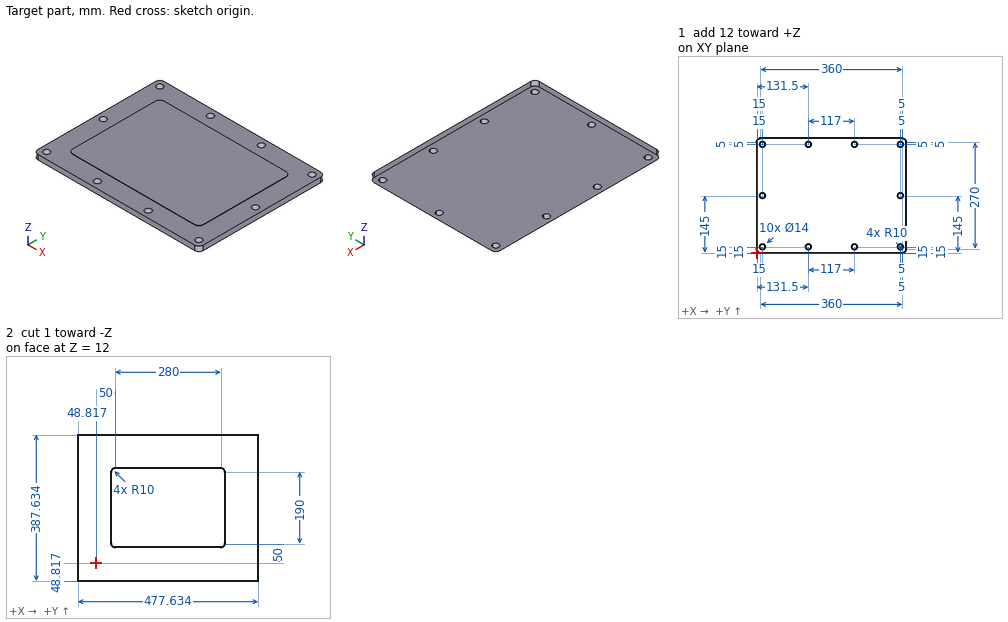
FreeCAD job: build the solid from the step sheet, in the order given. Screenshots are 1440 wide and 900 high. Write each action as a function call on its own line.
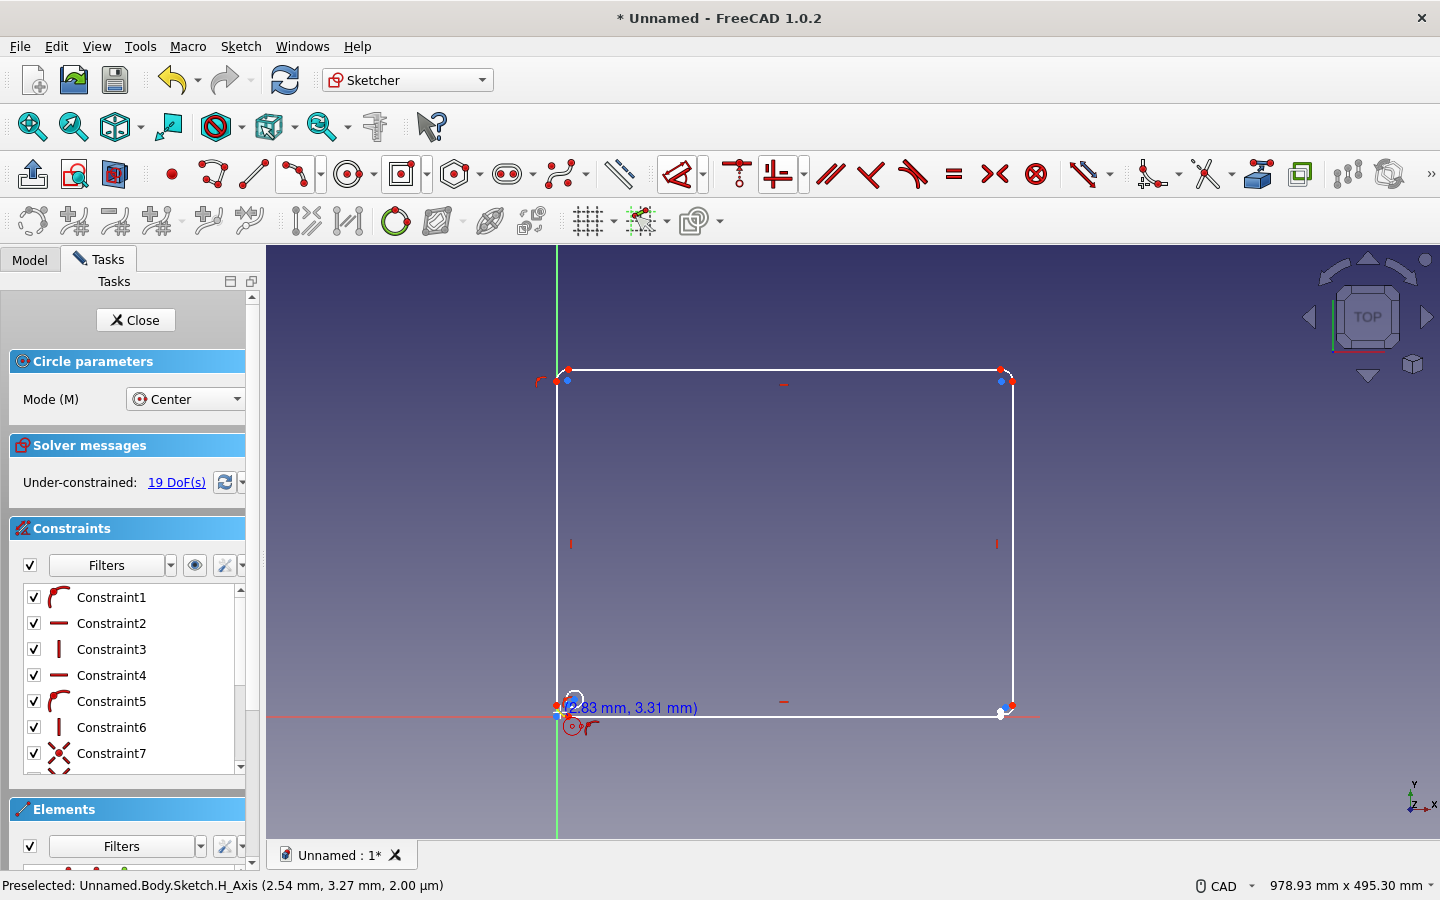
scroll(715, 699, up, 5)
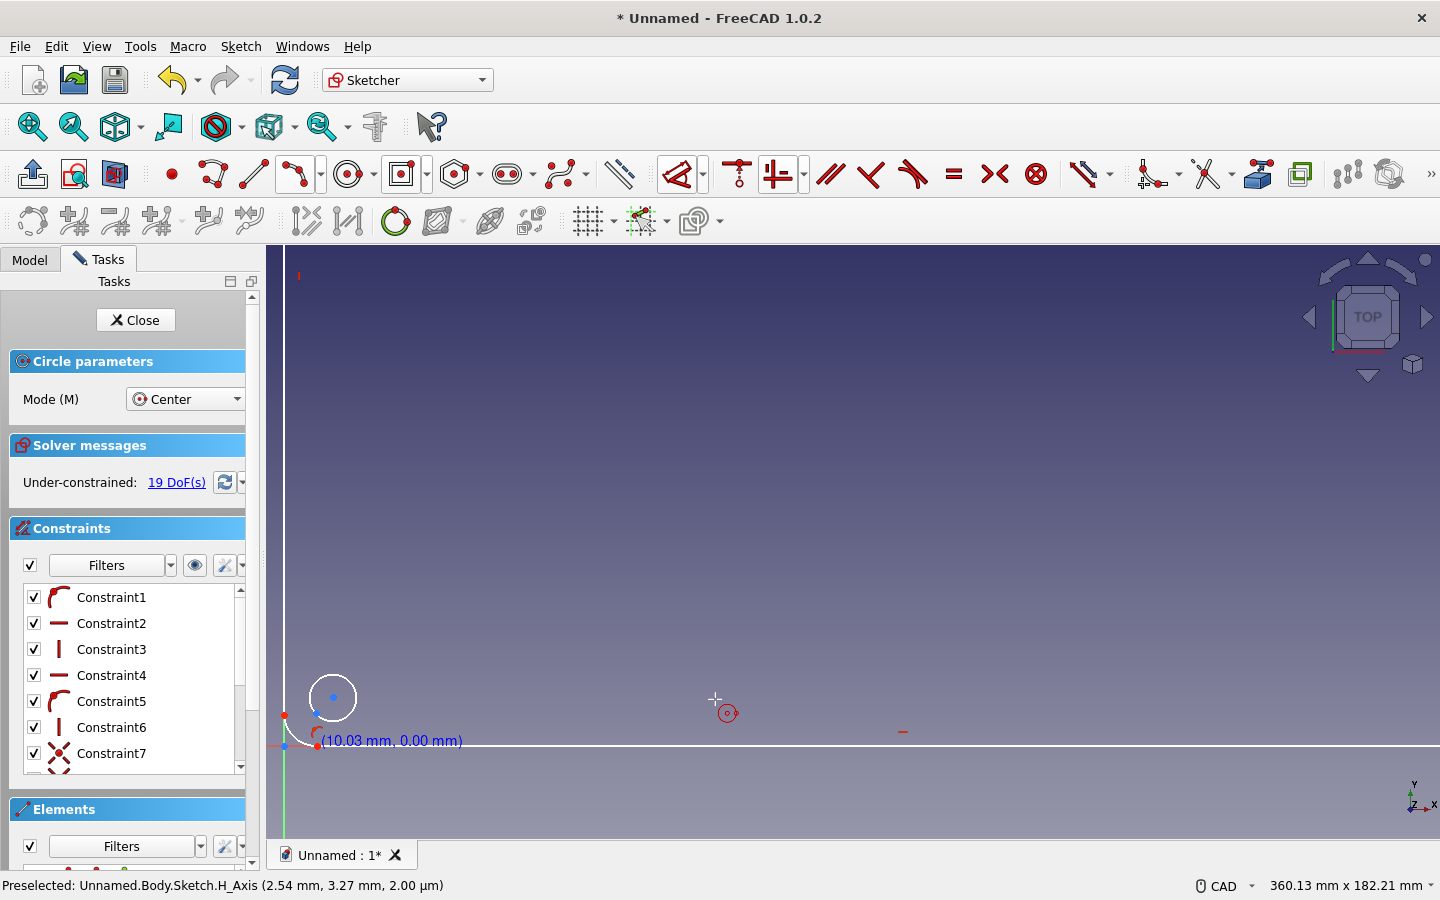
click(713, 697)
click(729, 681)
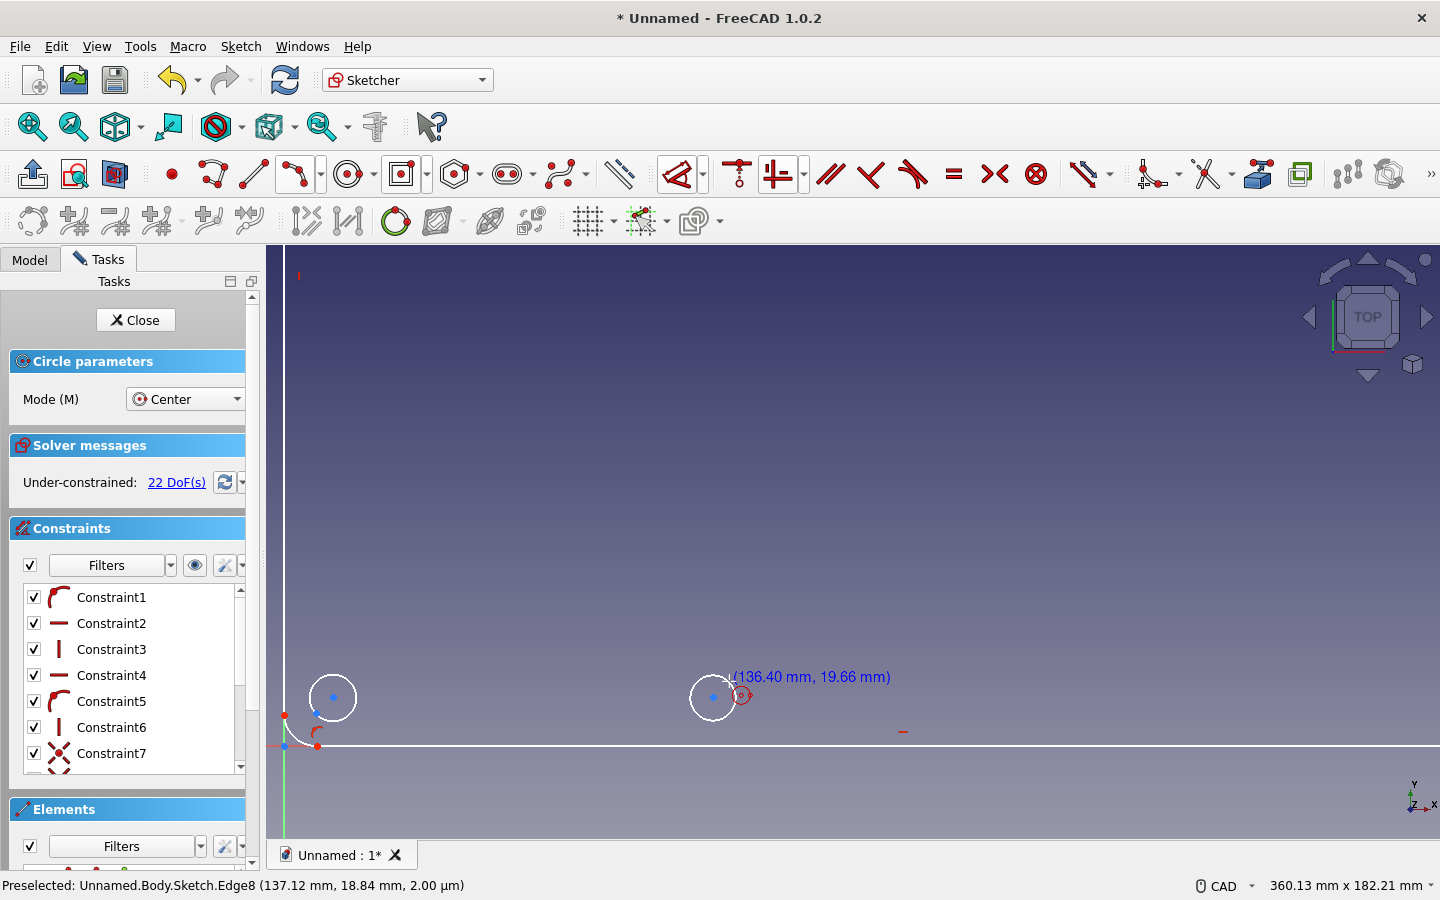
click(1094, 697)
click(1111, 681)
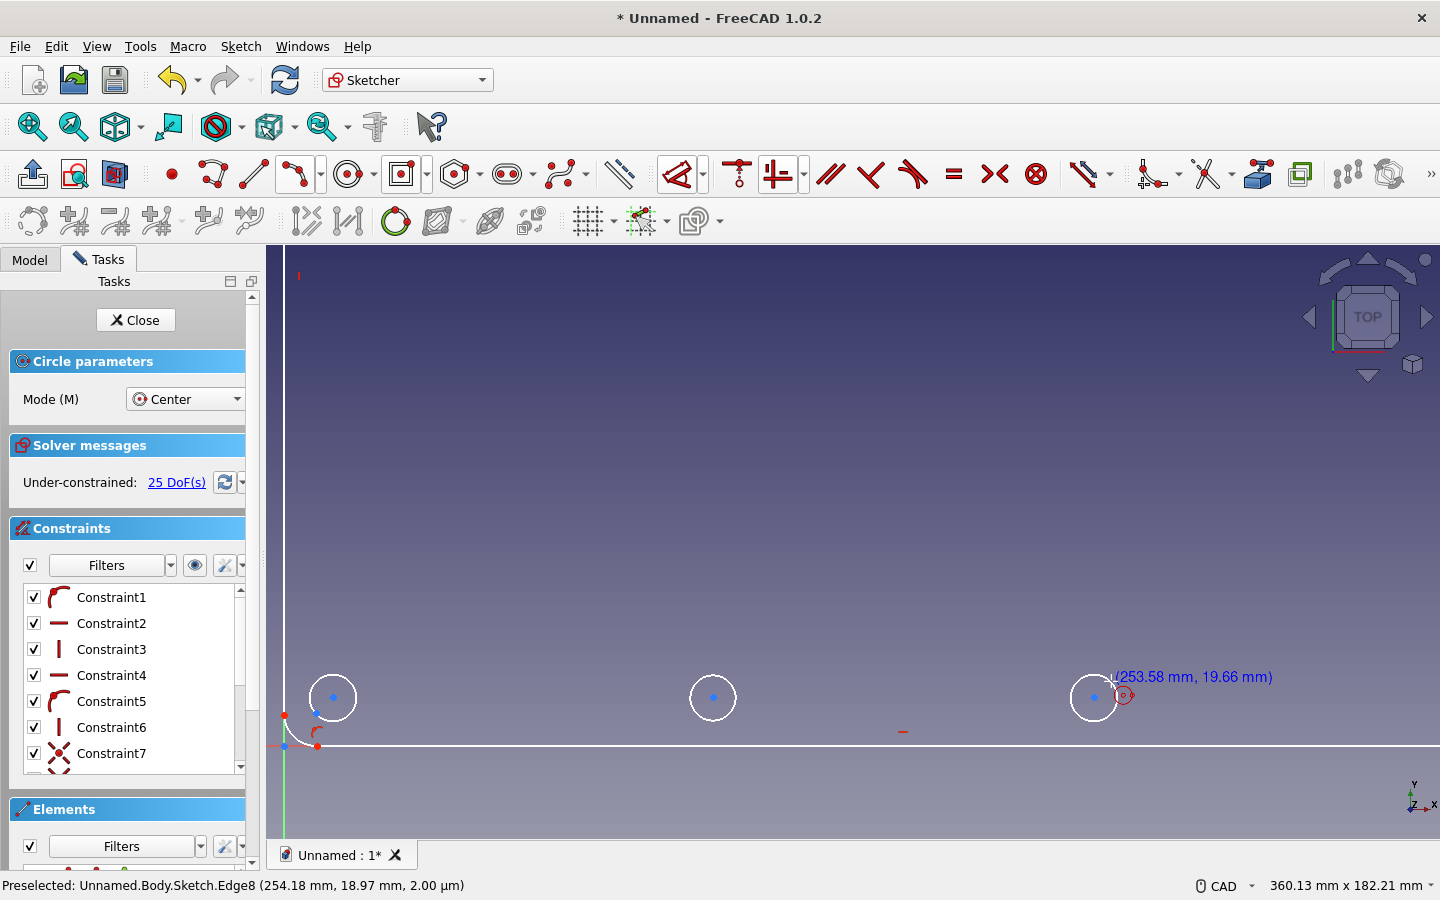
scroll(715, 698, down, 5)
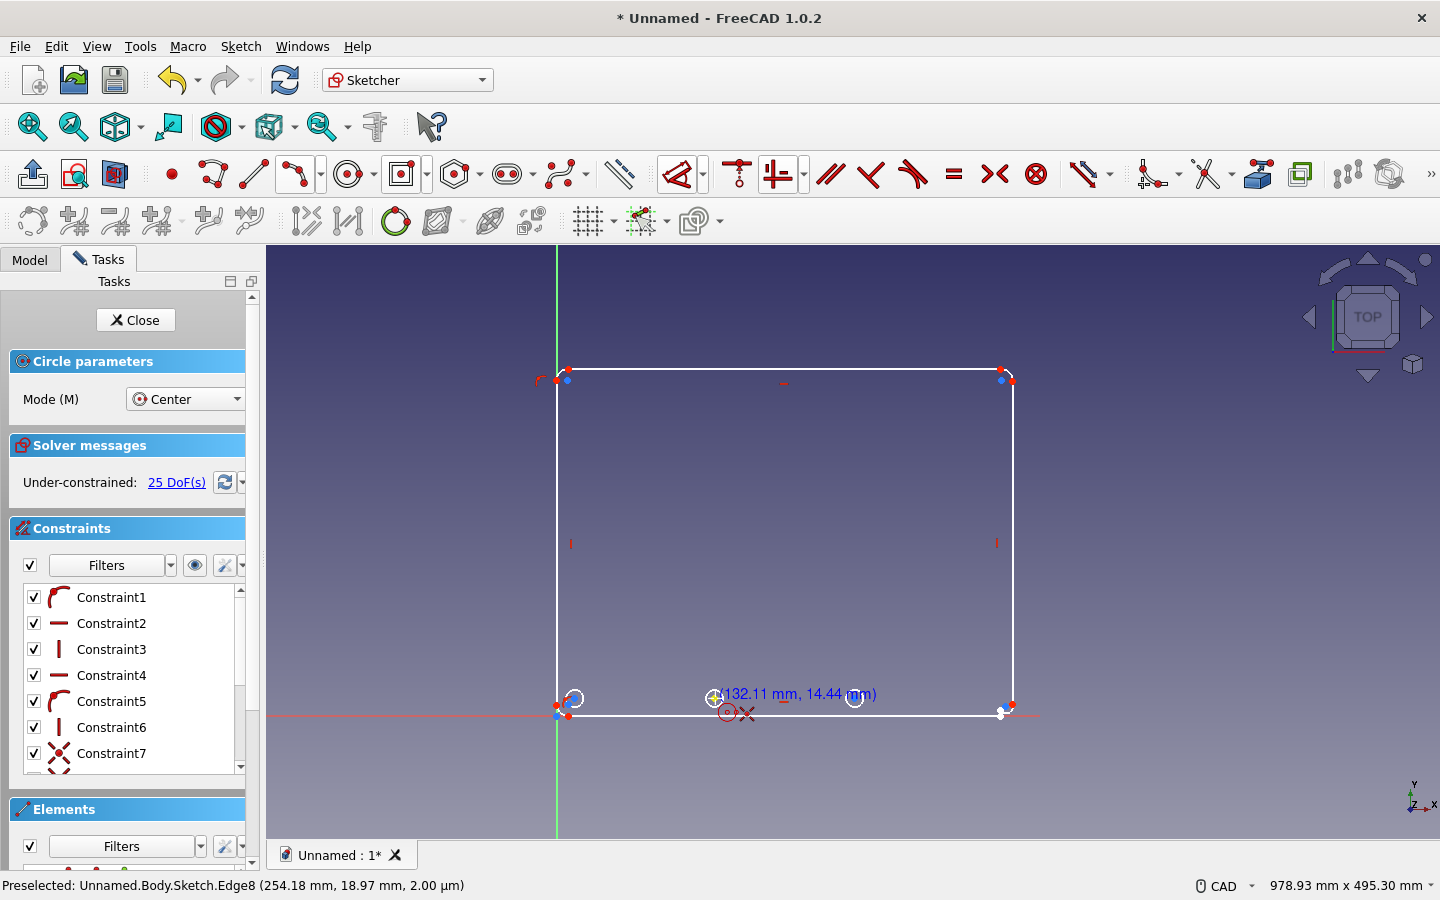
scroll(995, 698, up, 5)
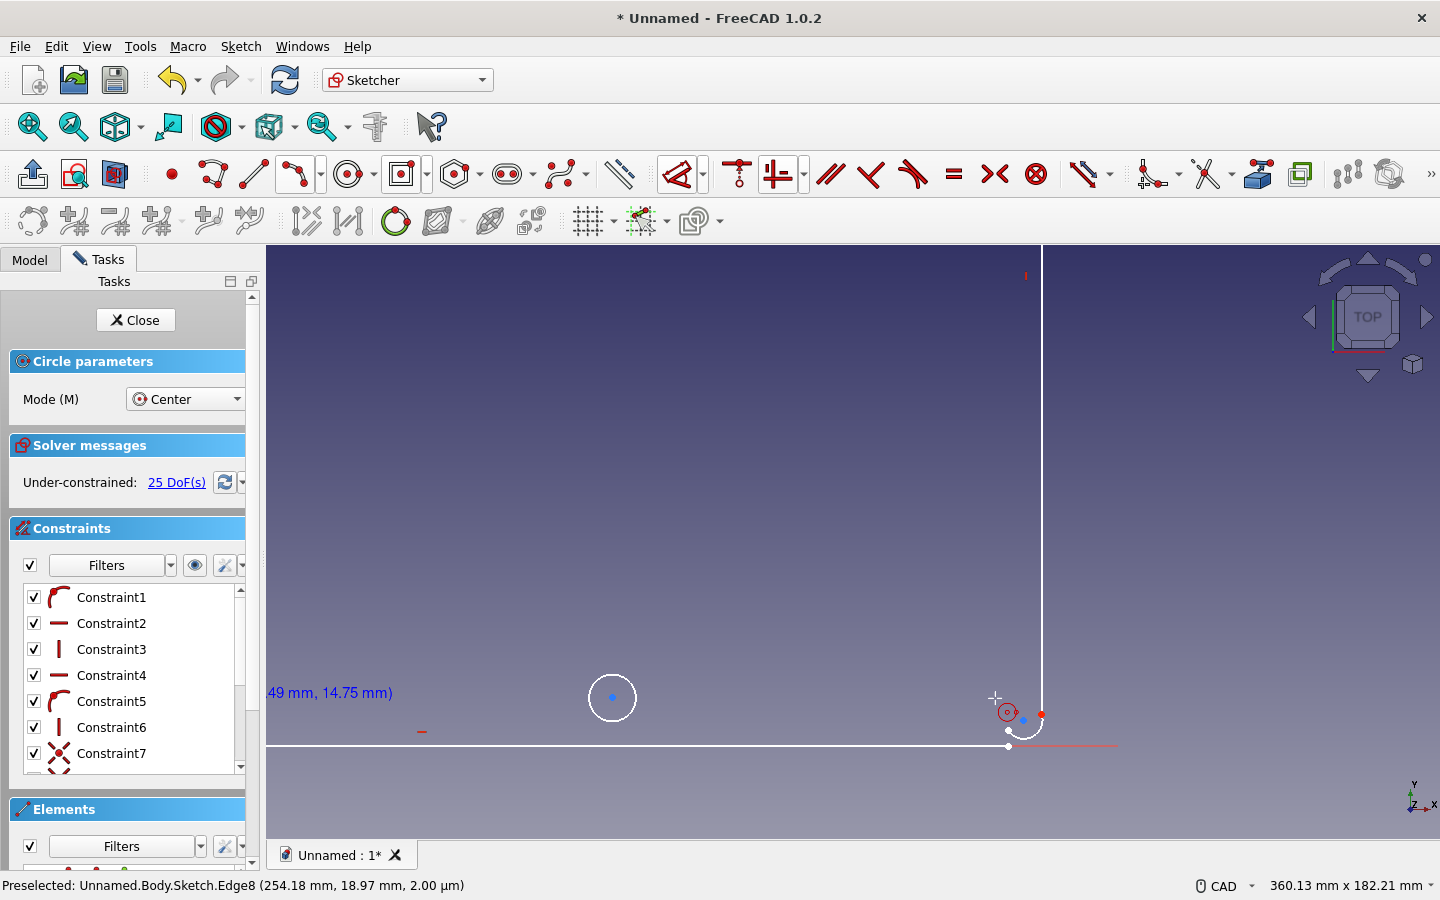
click(993, 697)
click(1009, 681)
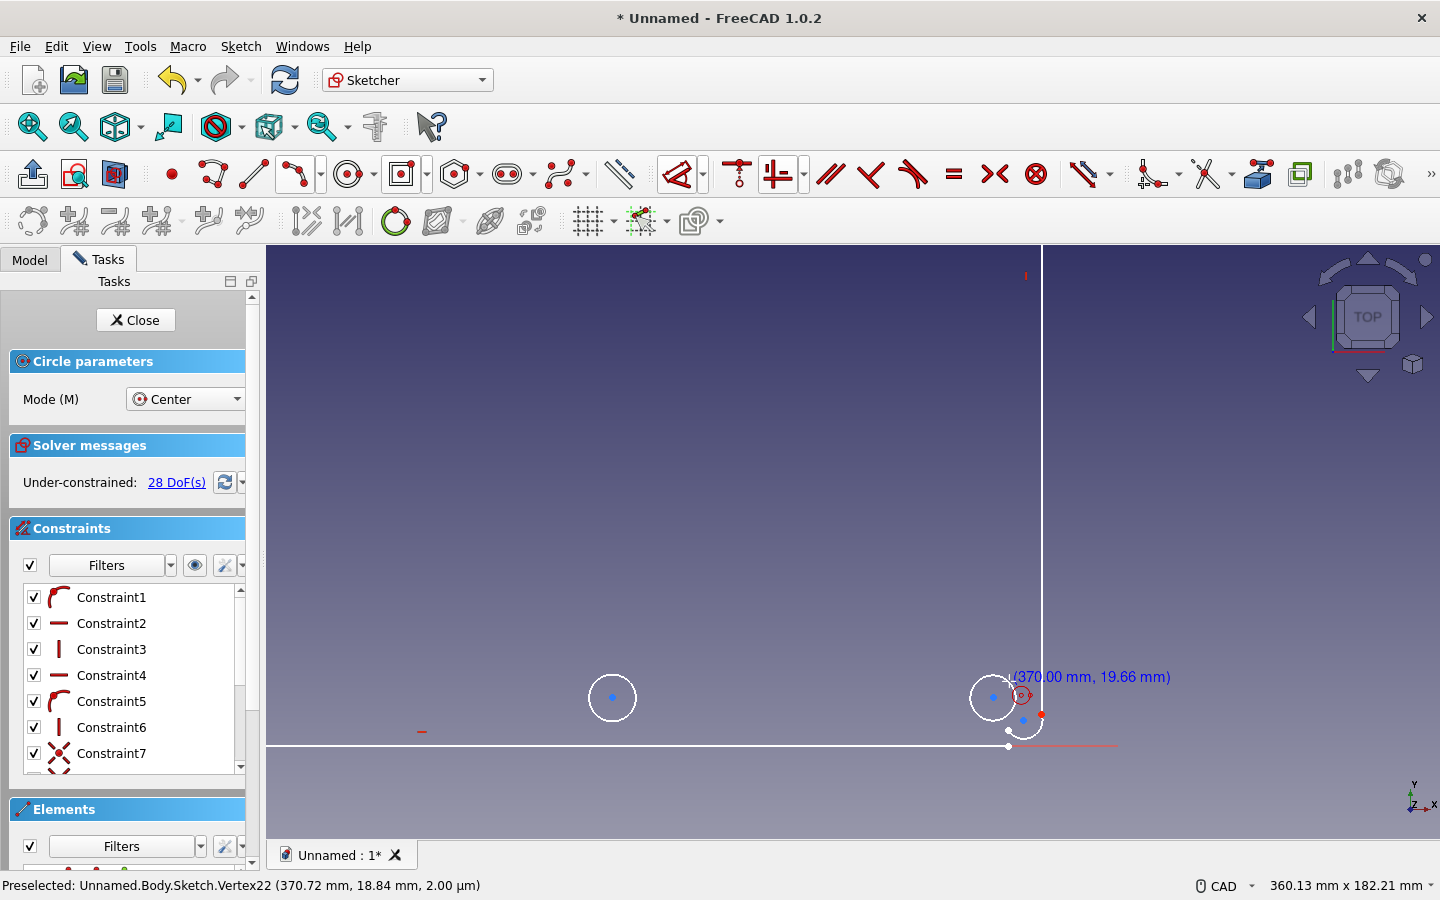
scroll(995, 698, down, 5)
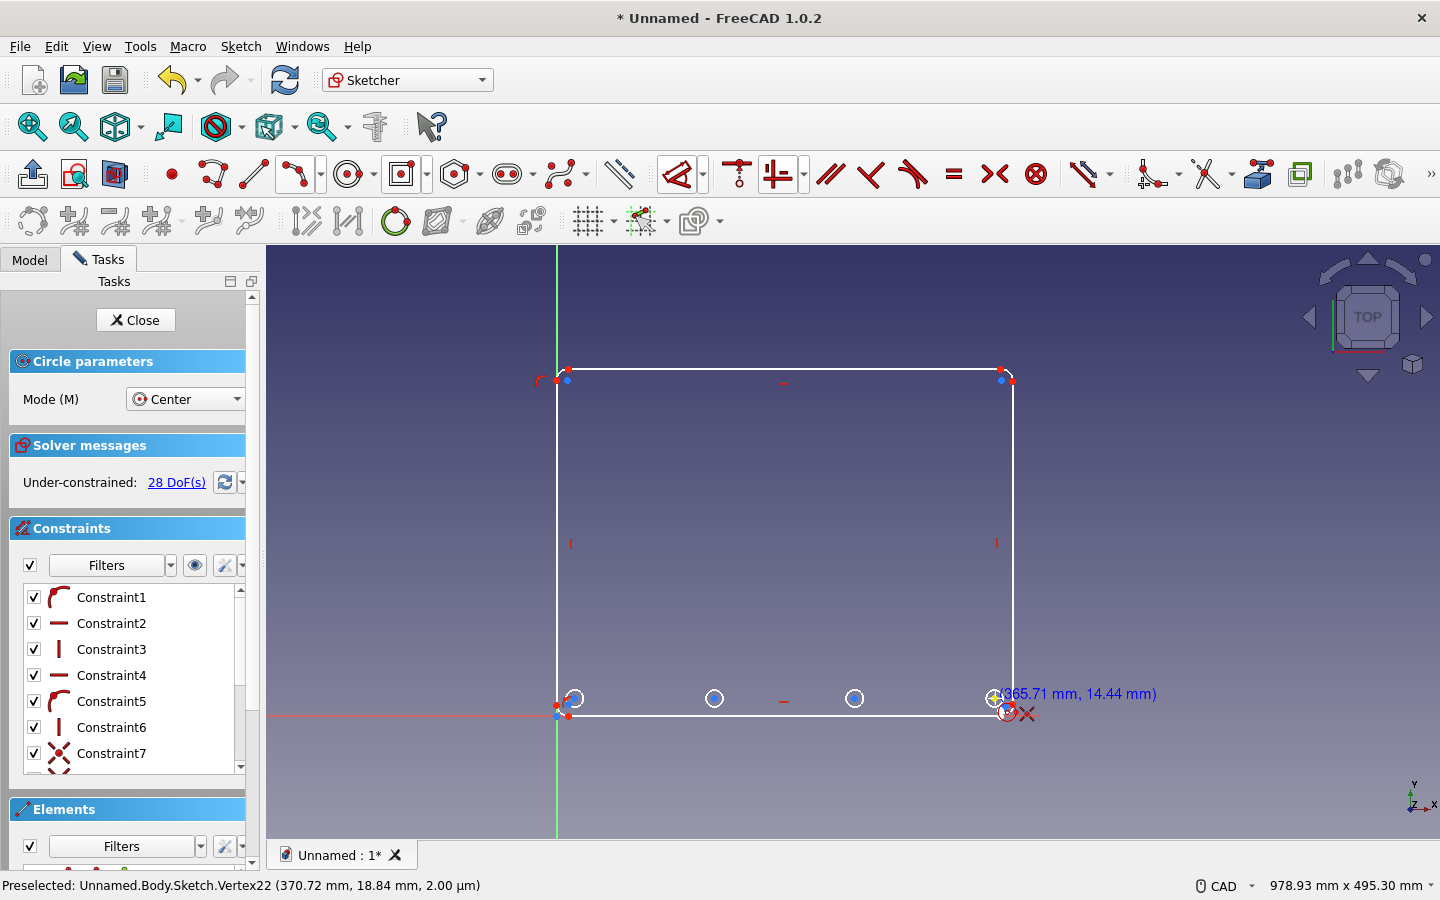
scroll(575, 542, up, 5)